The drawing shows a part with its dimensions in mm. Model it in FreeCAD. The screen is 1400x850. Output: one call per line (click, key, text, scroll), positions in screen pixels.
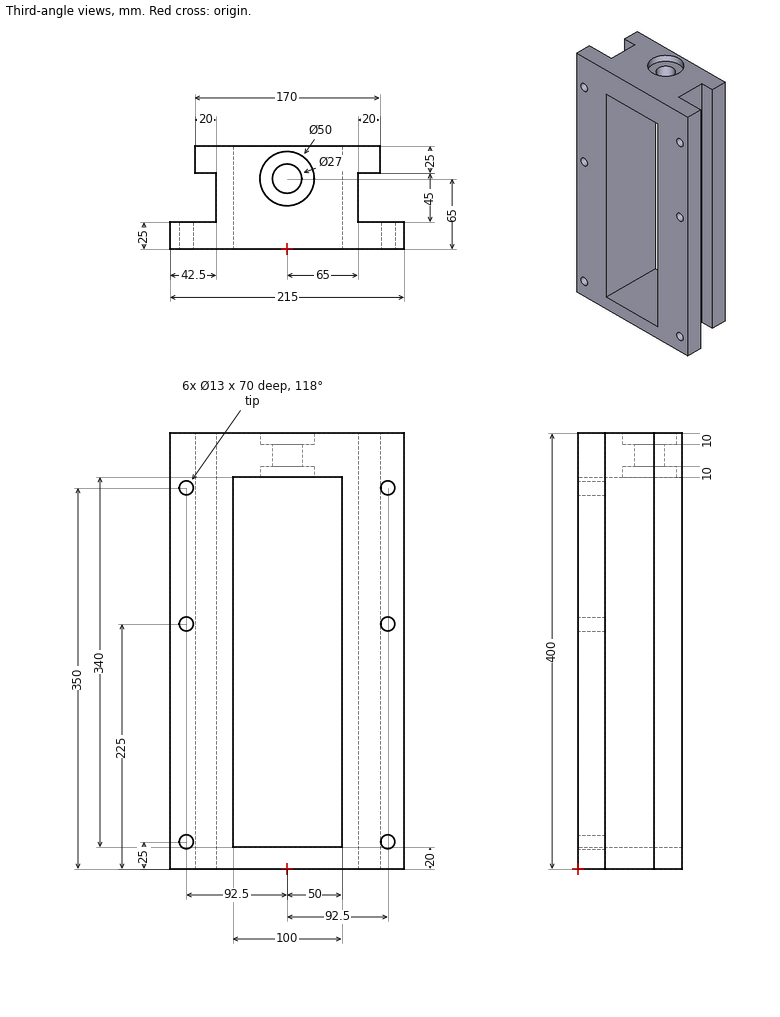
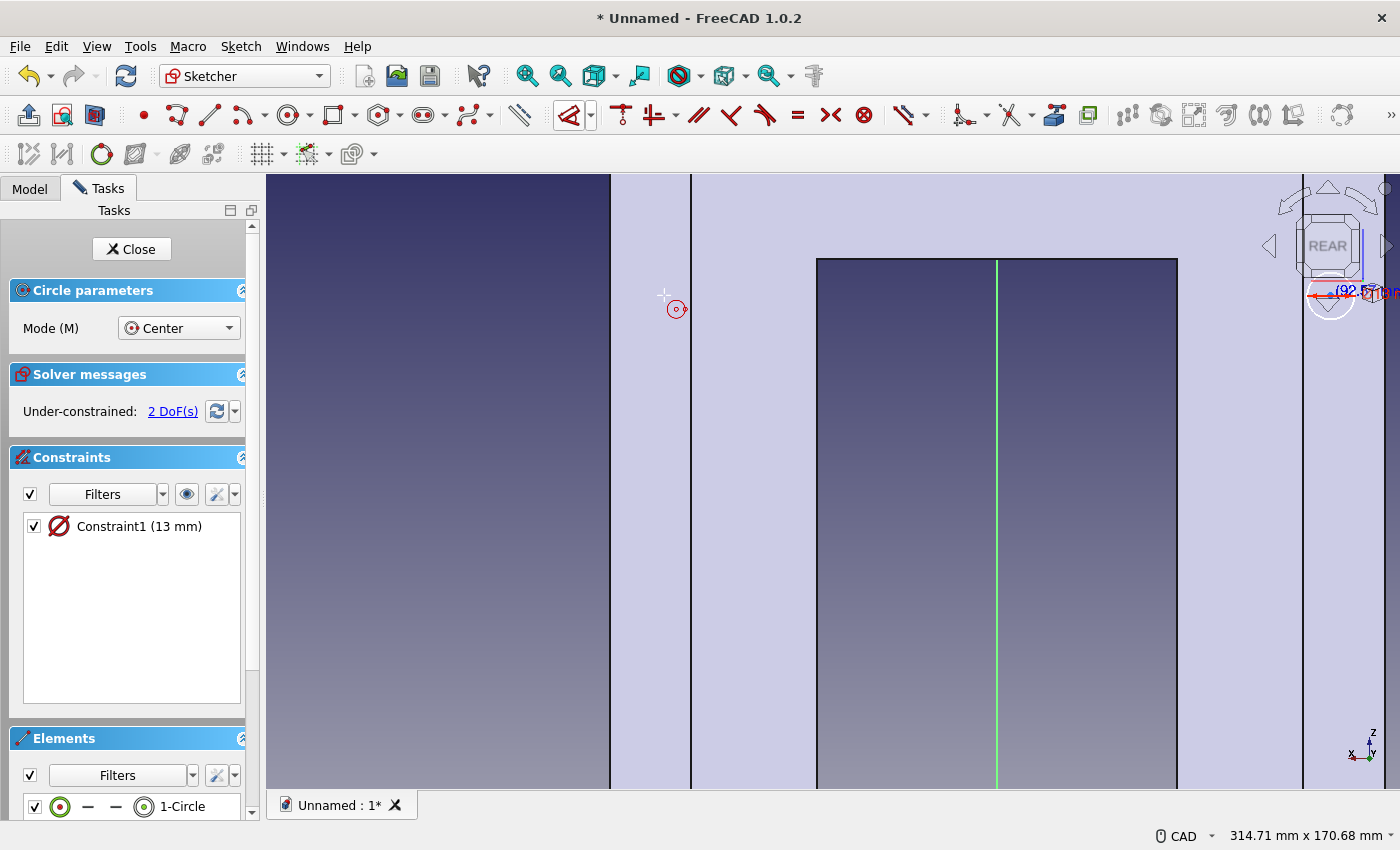
click(664, 295)
move(680, 279)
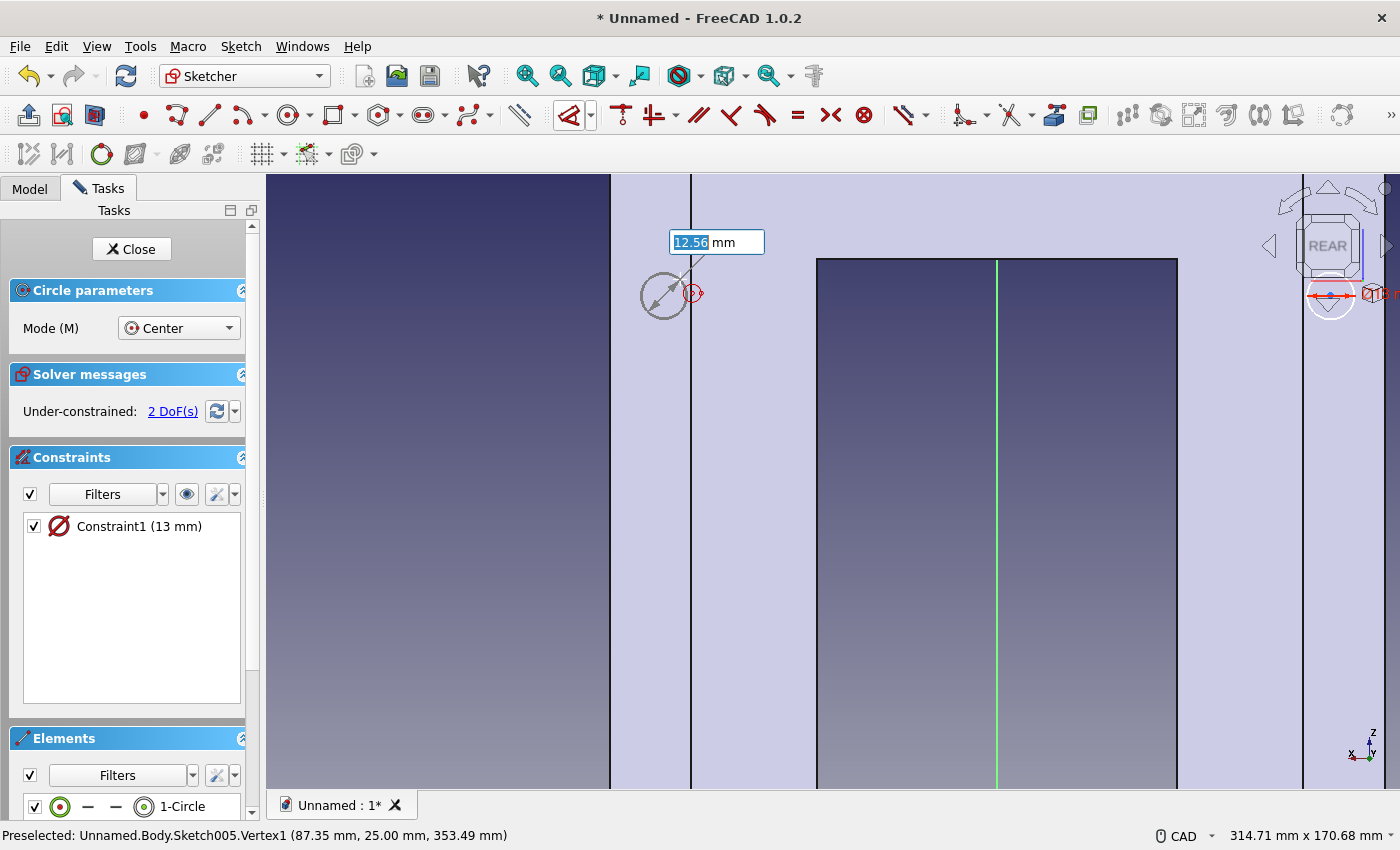
text(13)
key(Return)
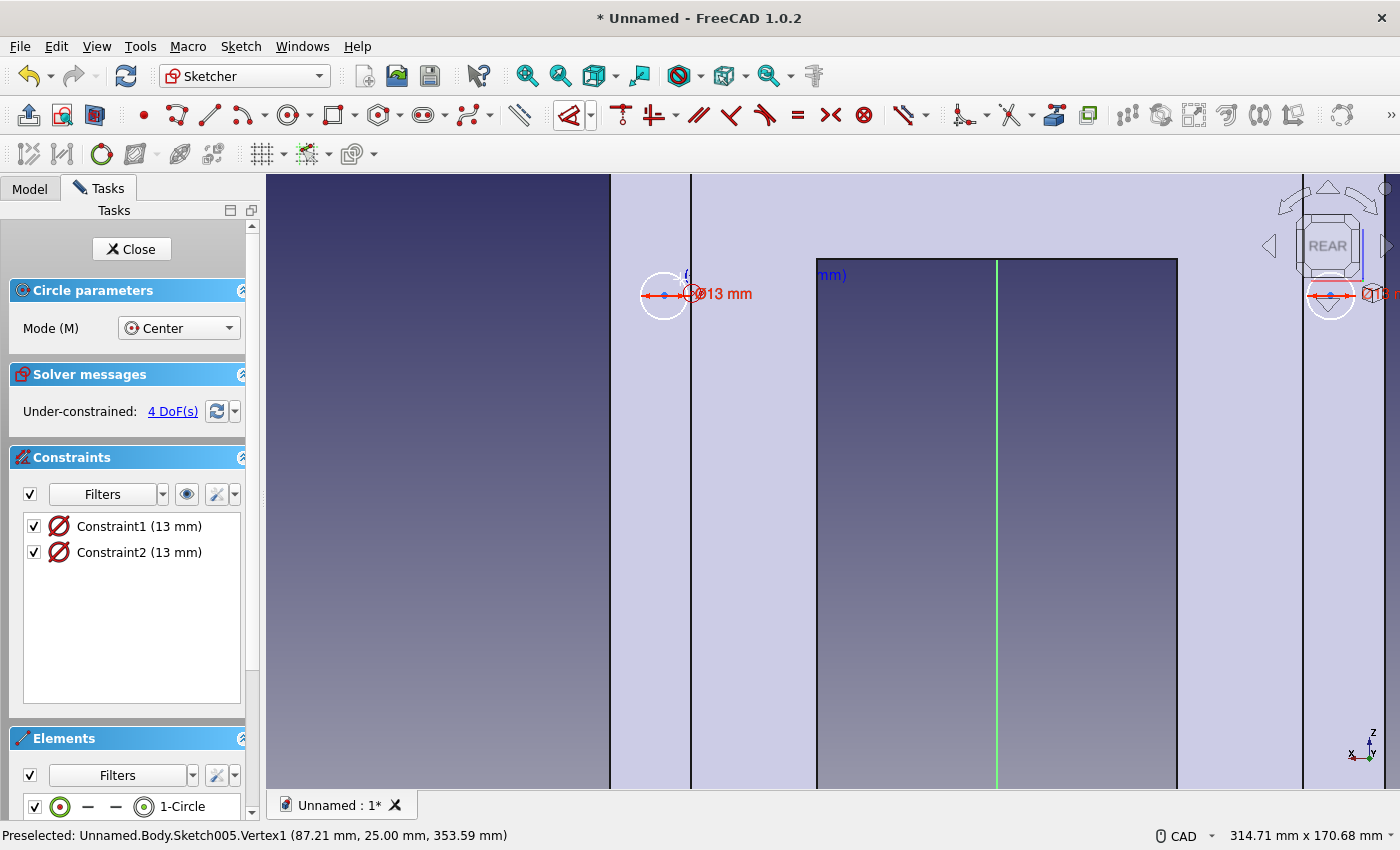
scroll(664, 295, down, 6)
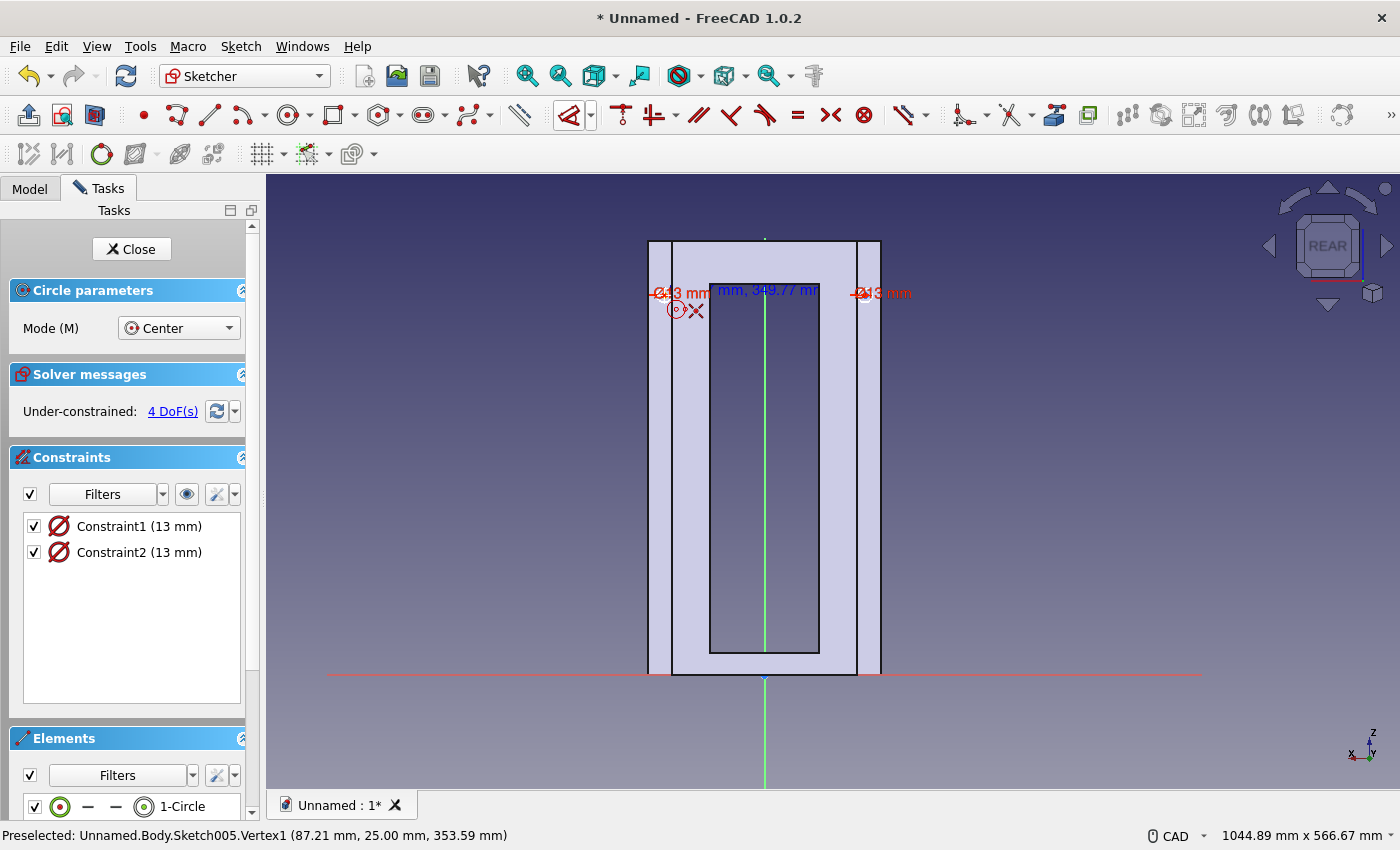
scroll(865, 431, up, 6)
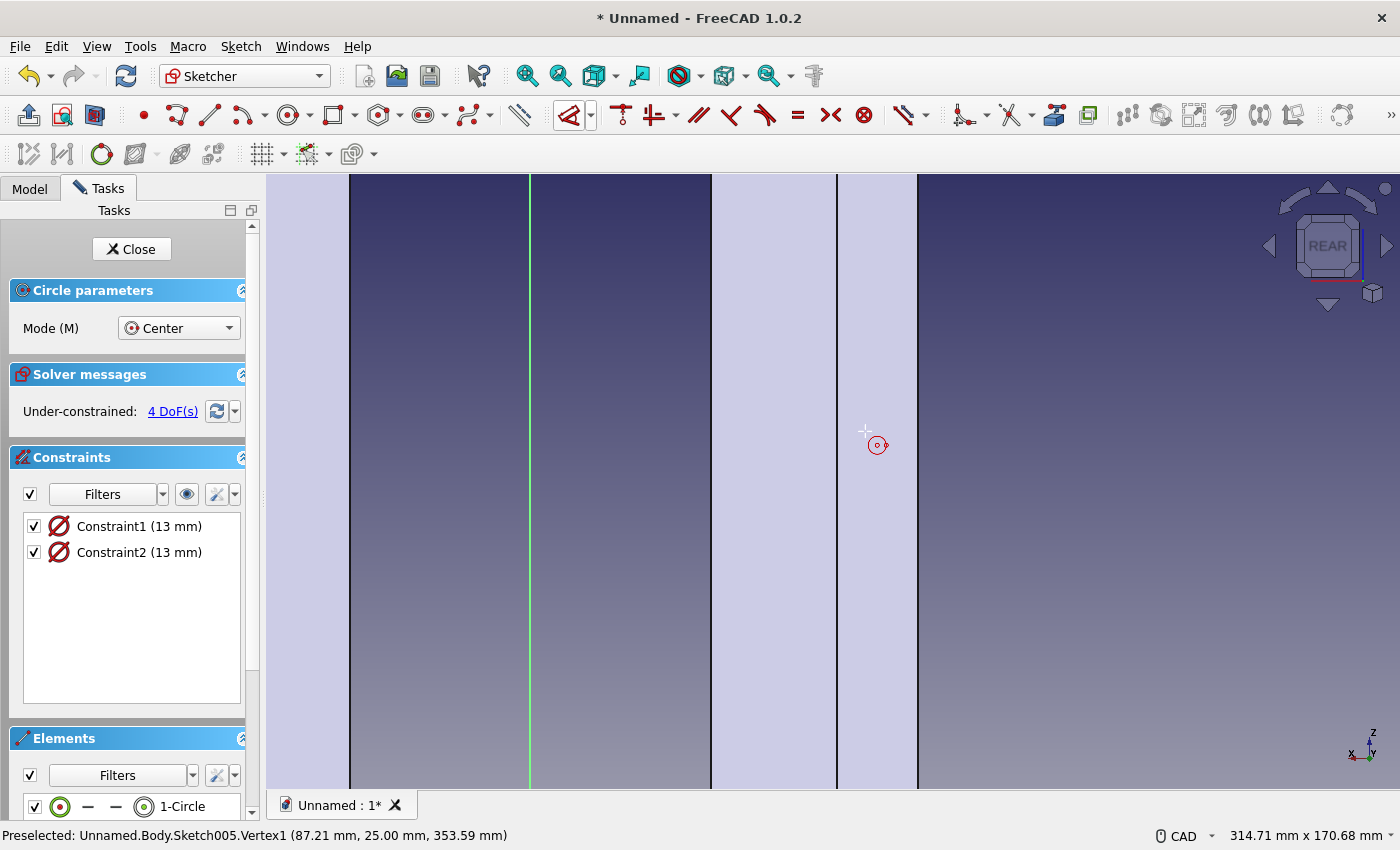
click(864, 430)
move(880, 413)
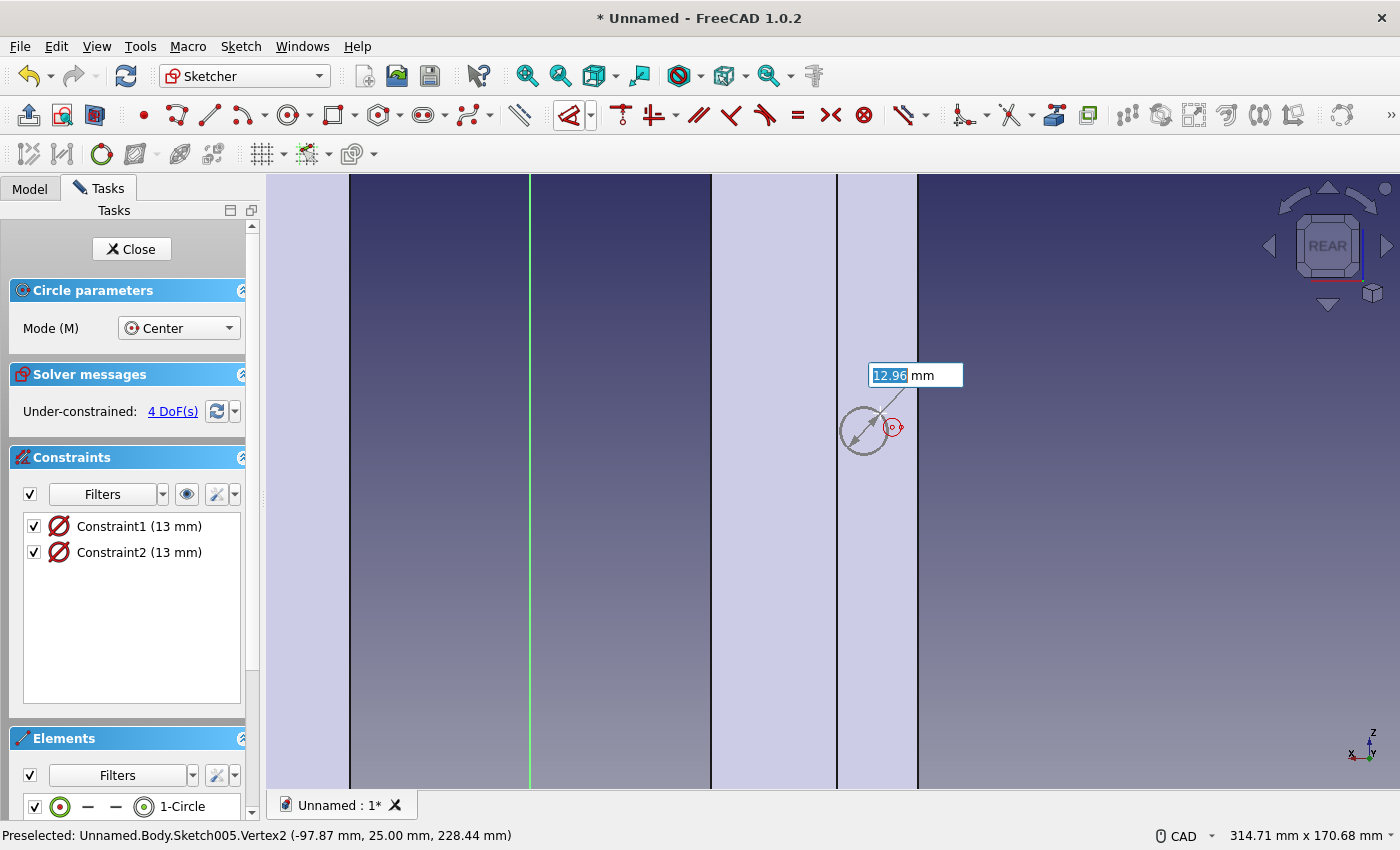
text(13)
key(Return)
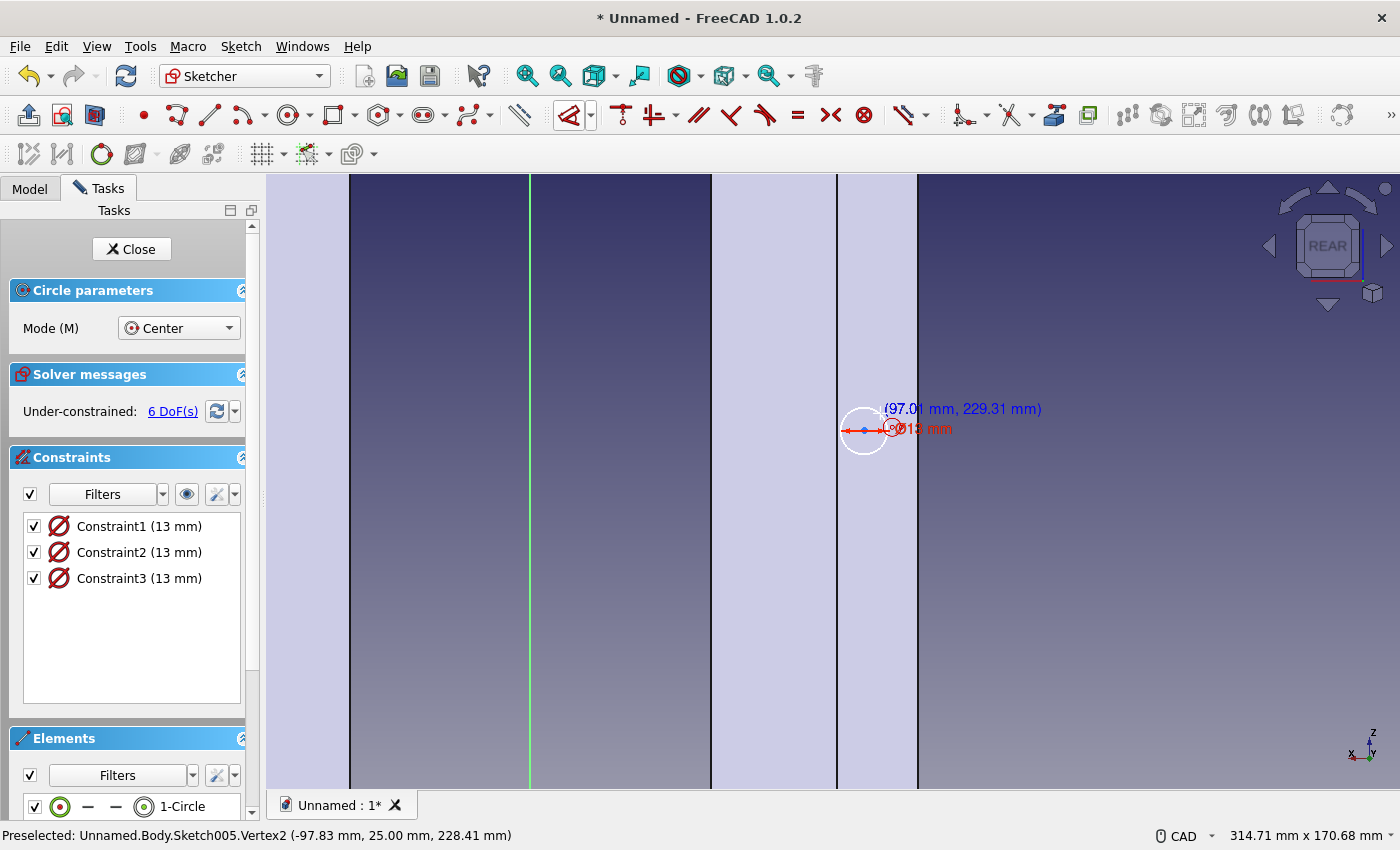
scroll(865, 431, down, 6)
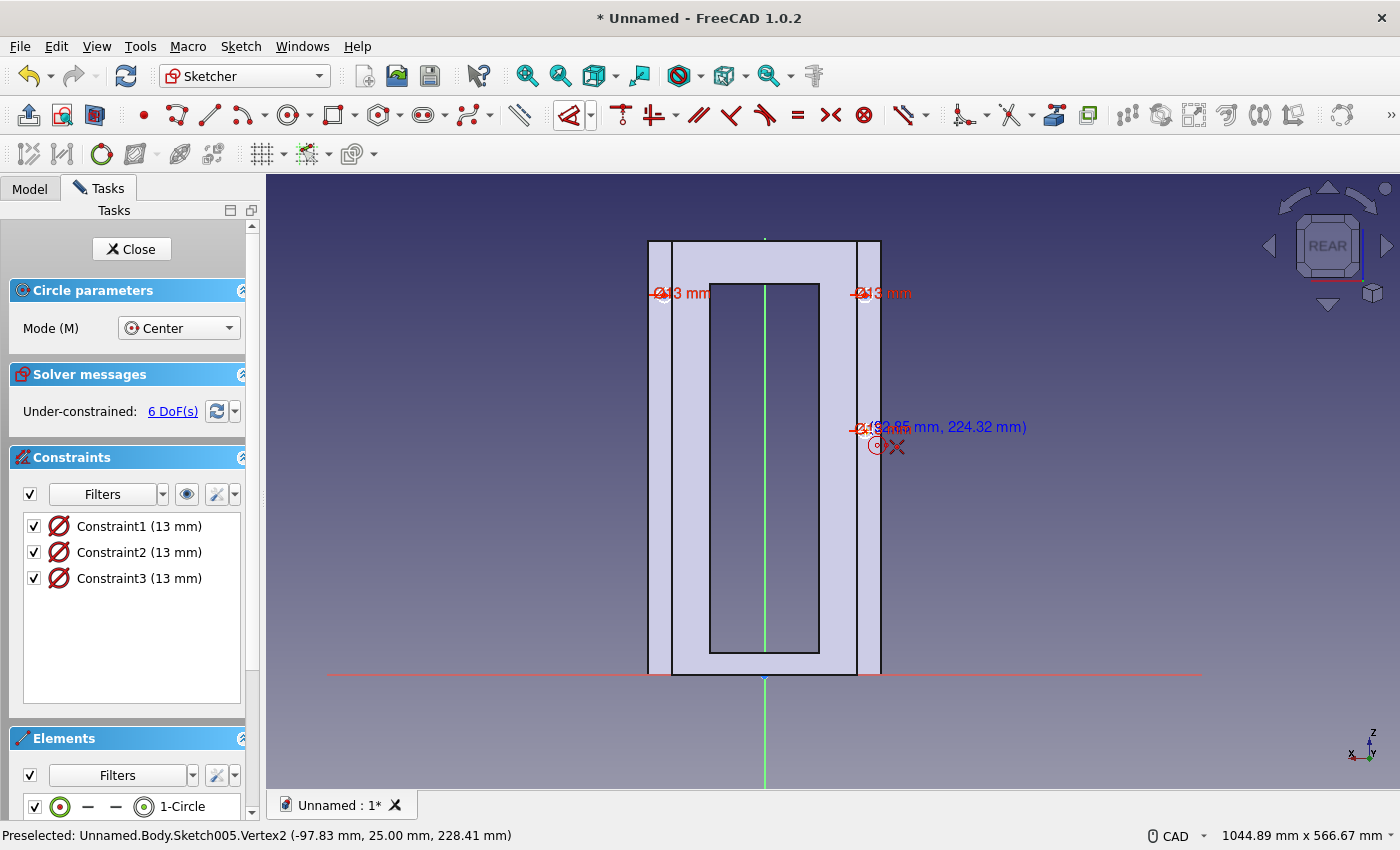
scroll(664, 431, up, 6)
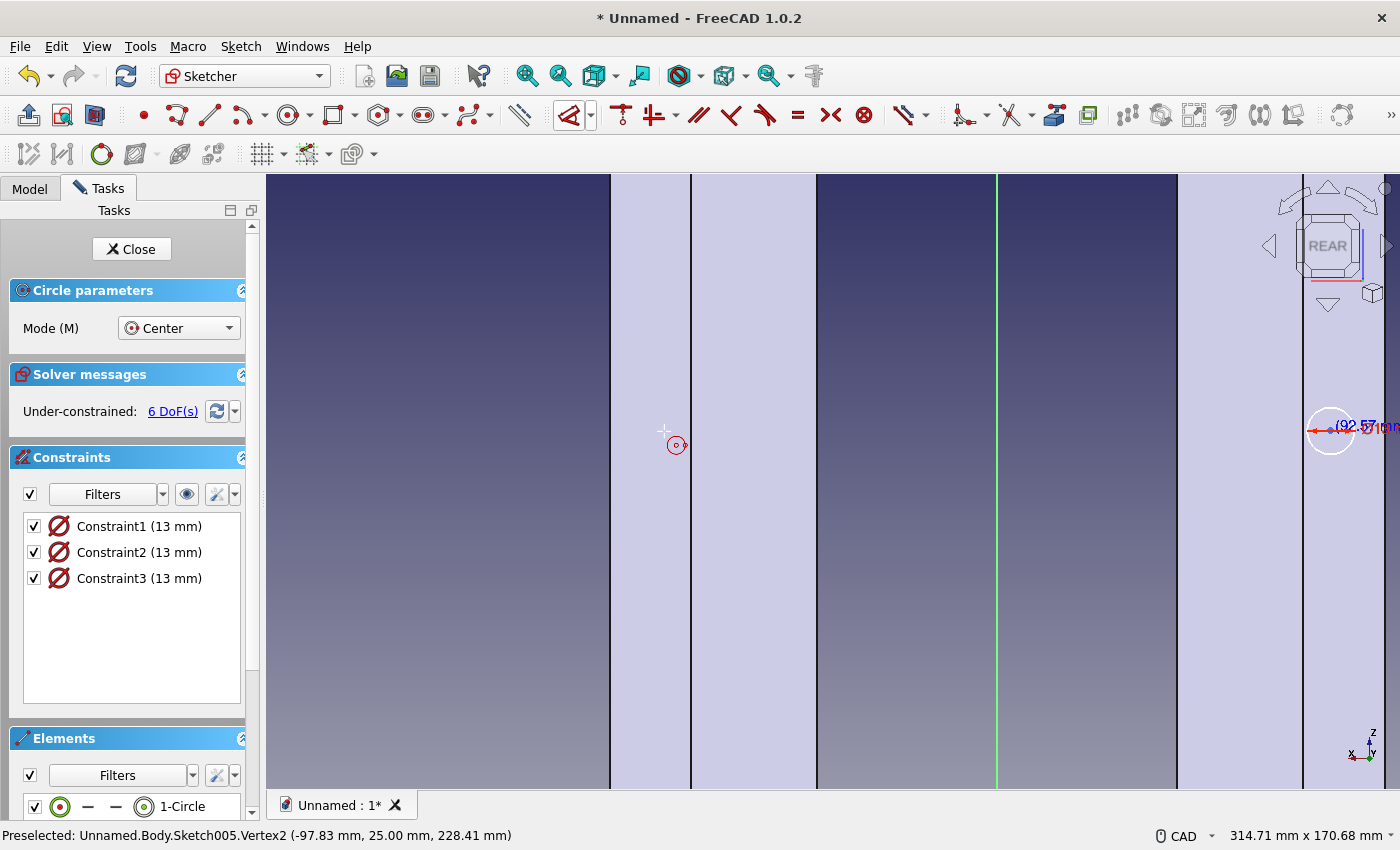
click(664, 430)
move(680, 413)